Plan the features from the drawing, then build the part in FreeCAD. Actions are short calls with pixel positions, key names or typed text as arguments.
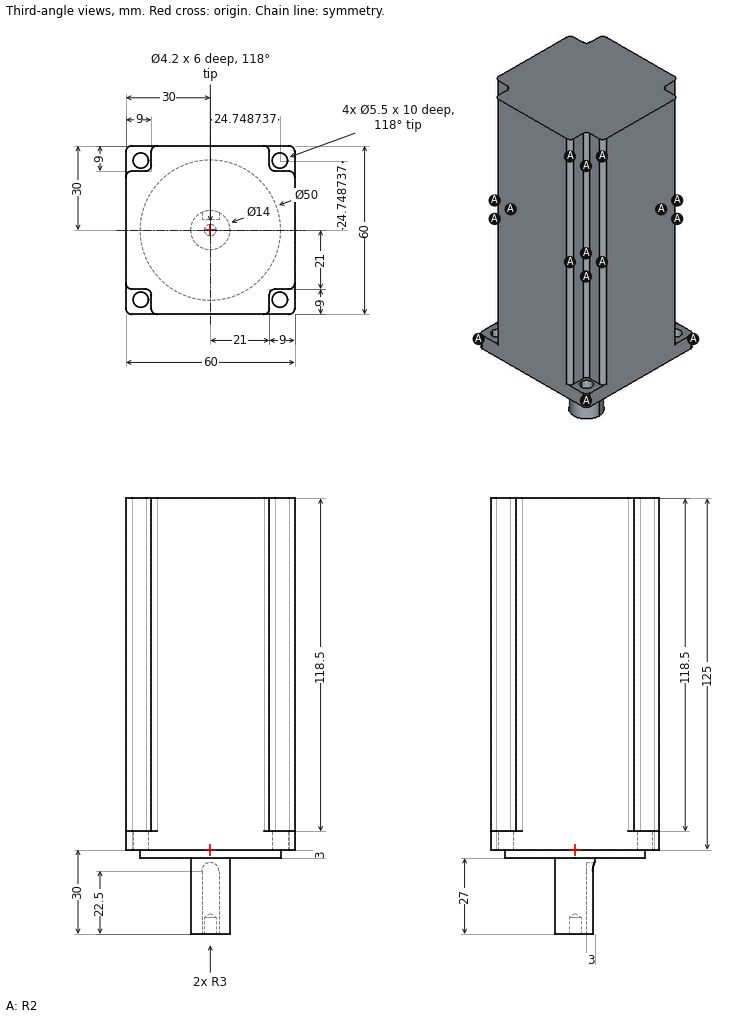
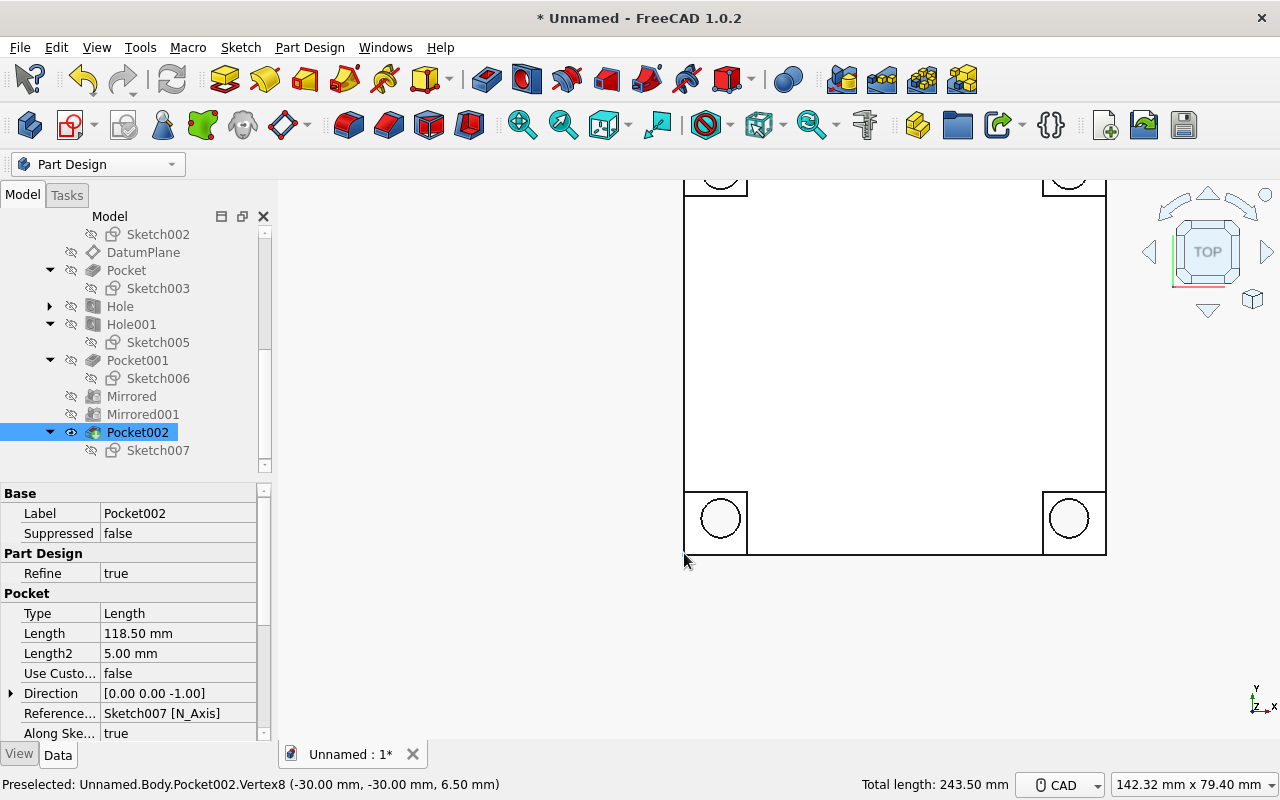
click(524, 126)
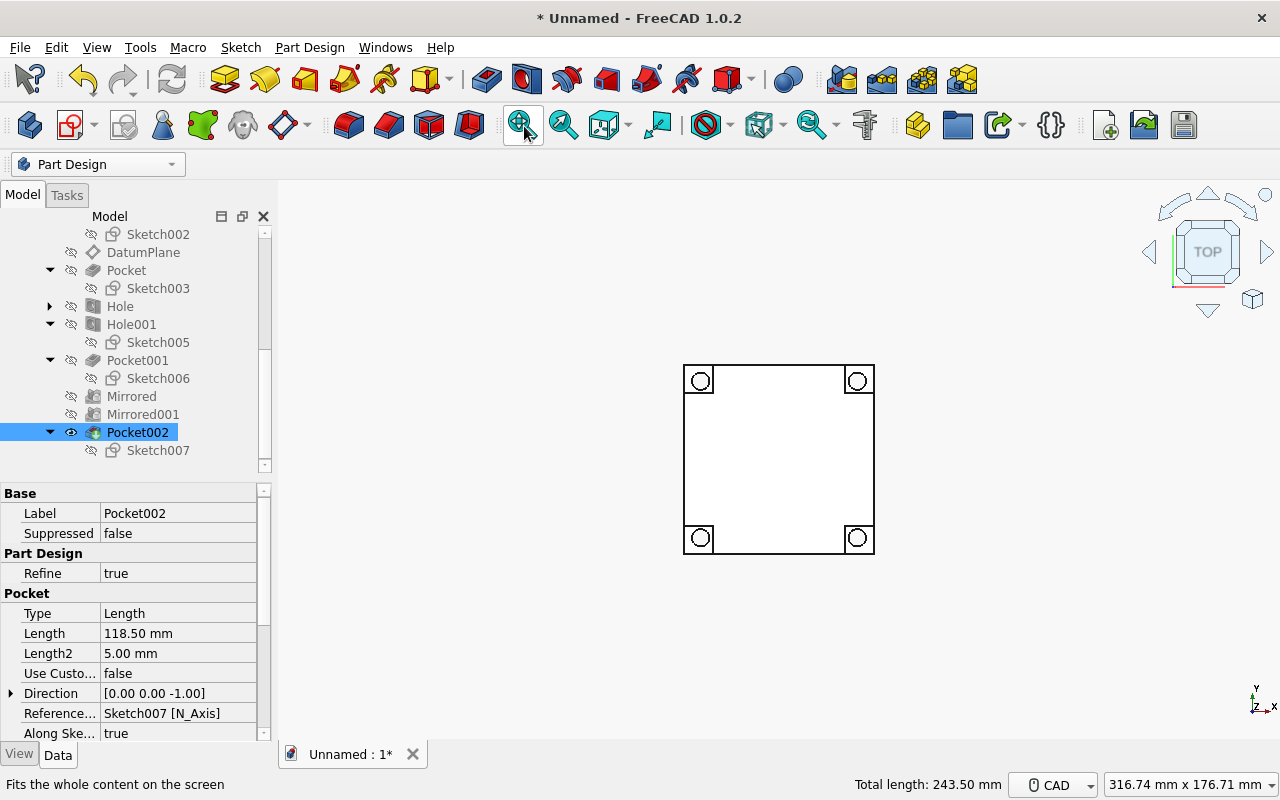
key(0)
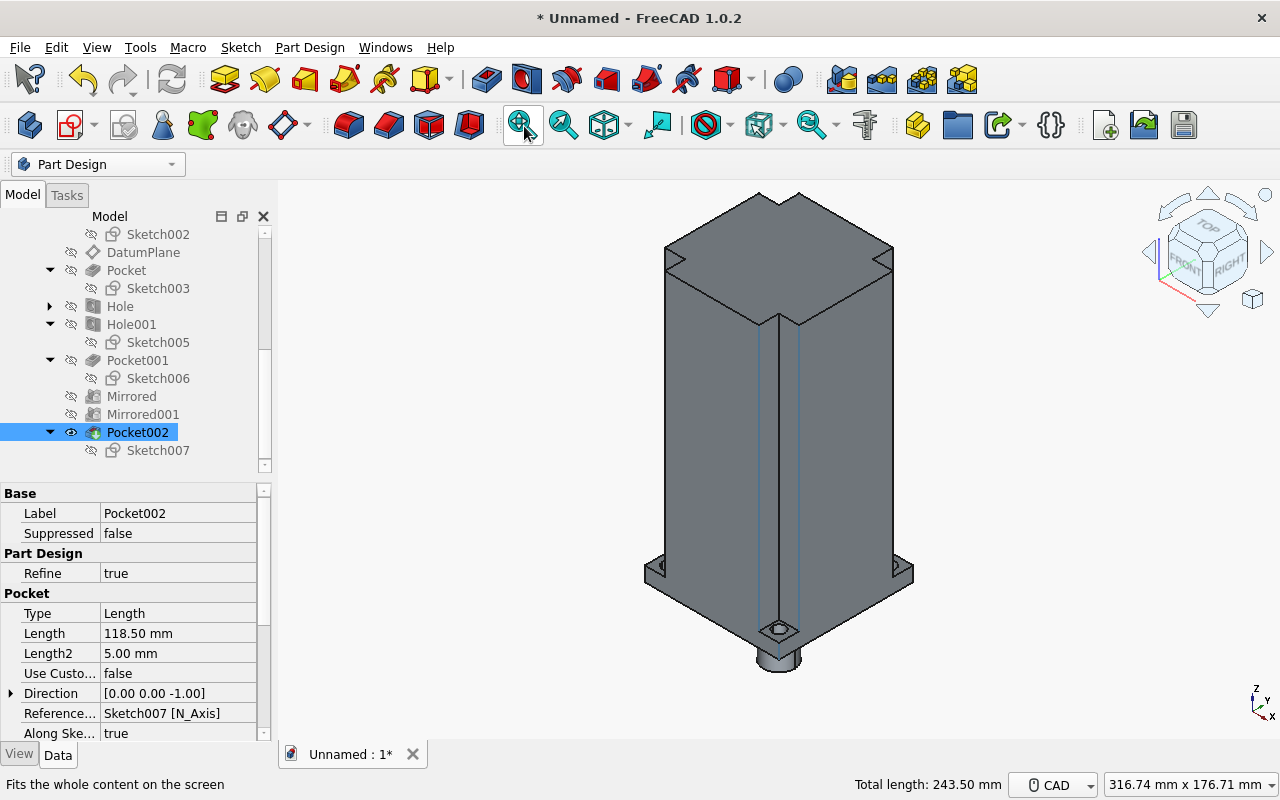
scroll(645, 573, up, 4)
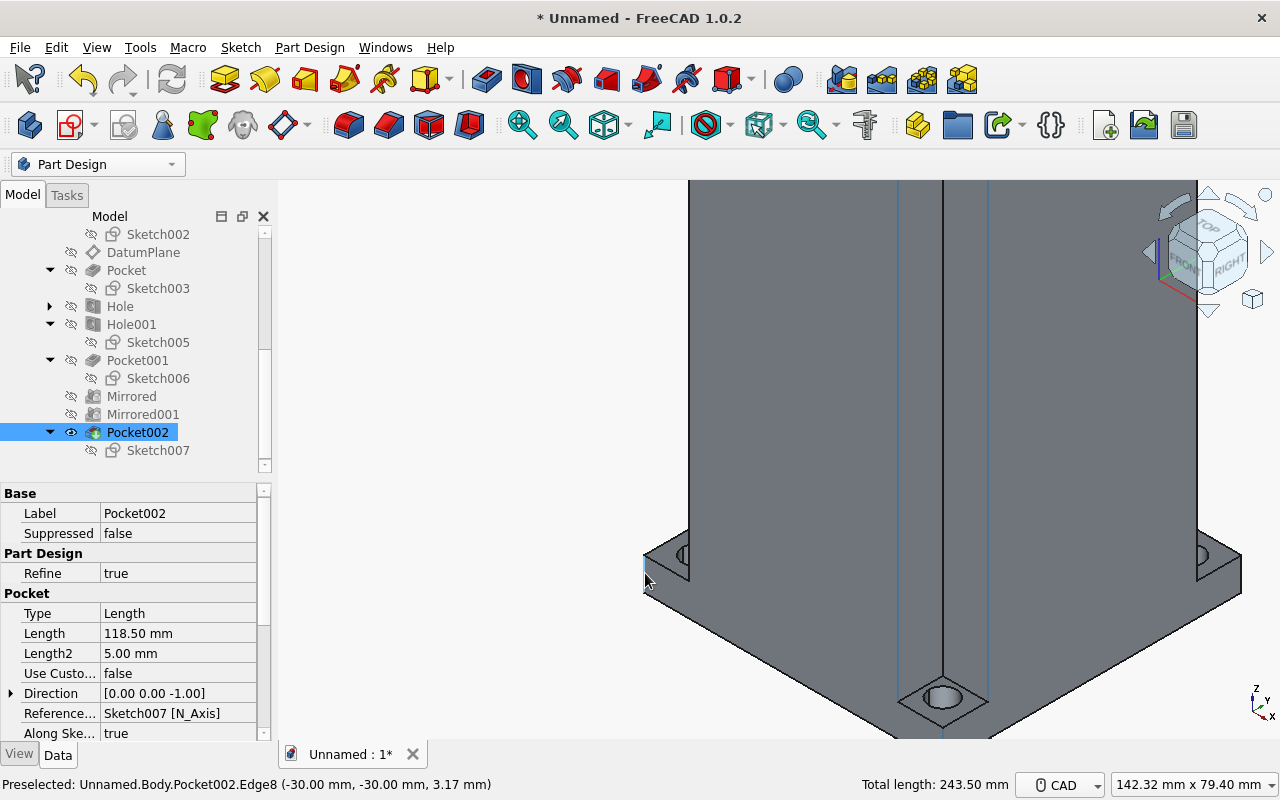
click(524, 126)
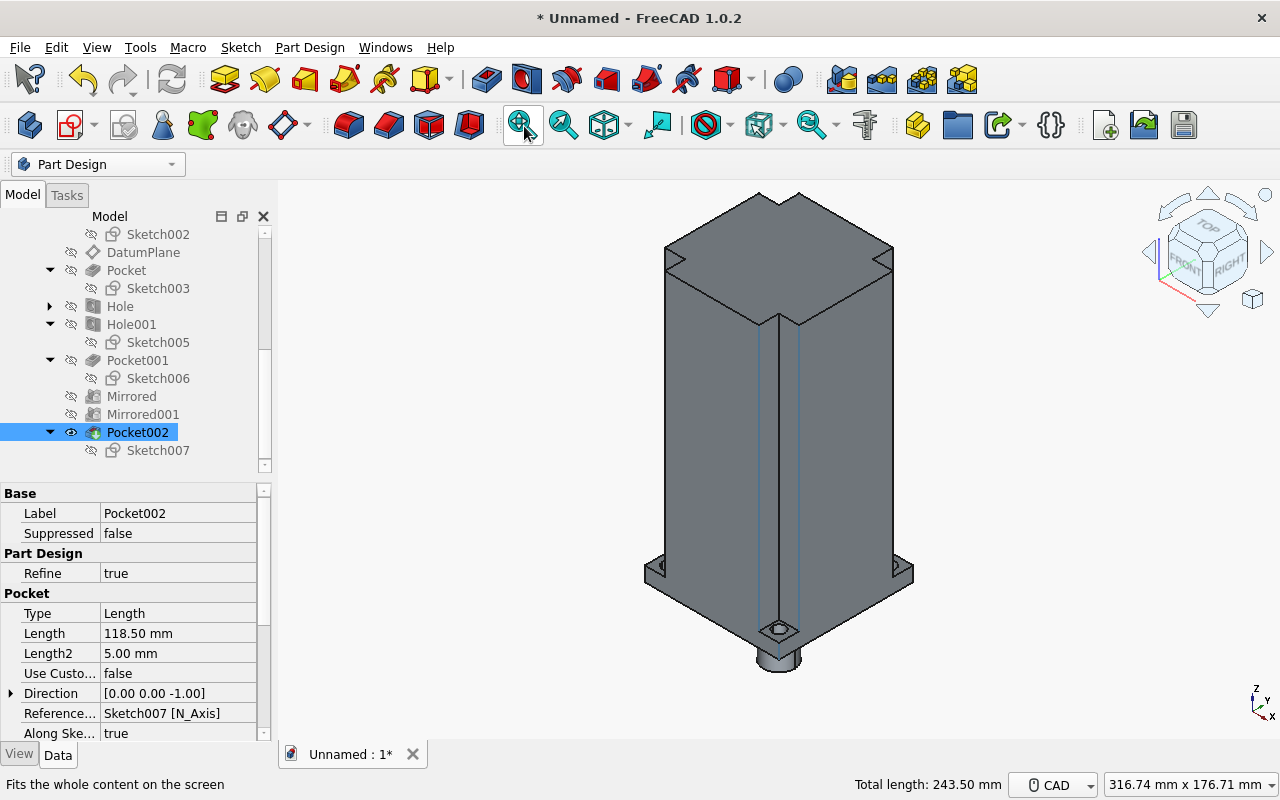
key(1)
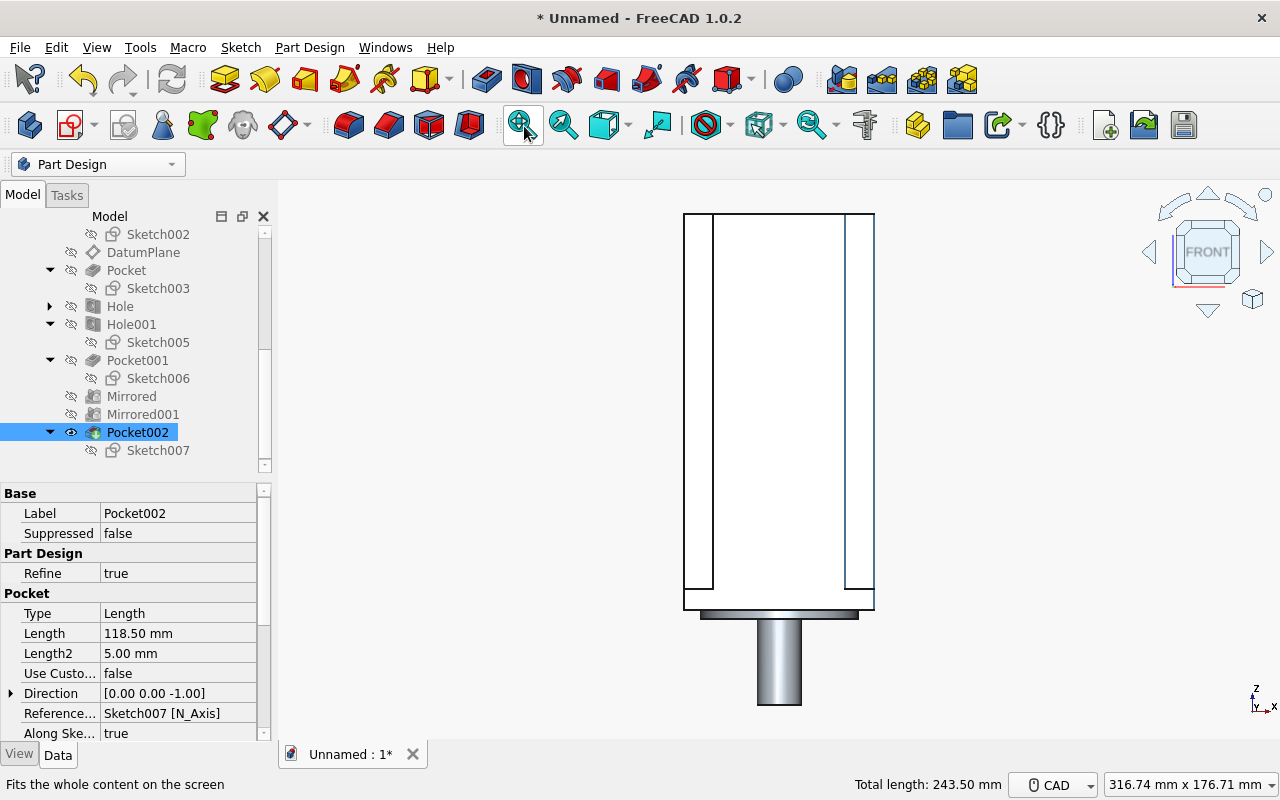
click(684, 598, ctrl)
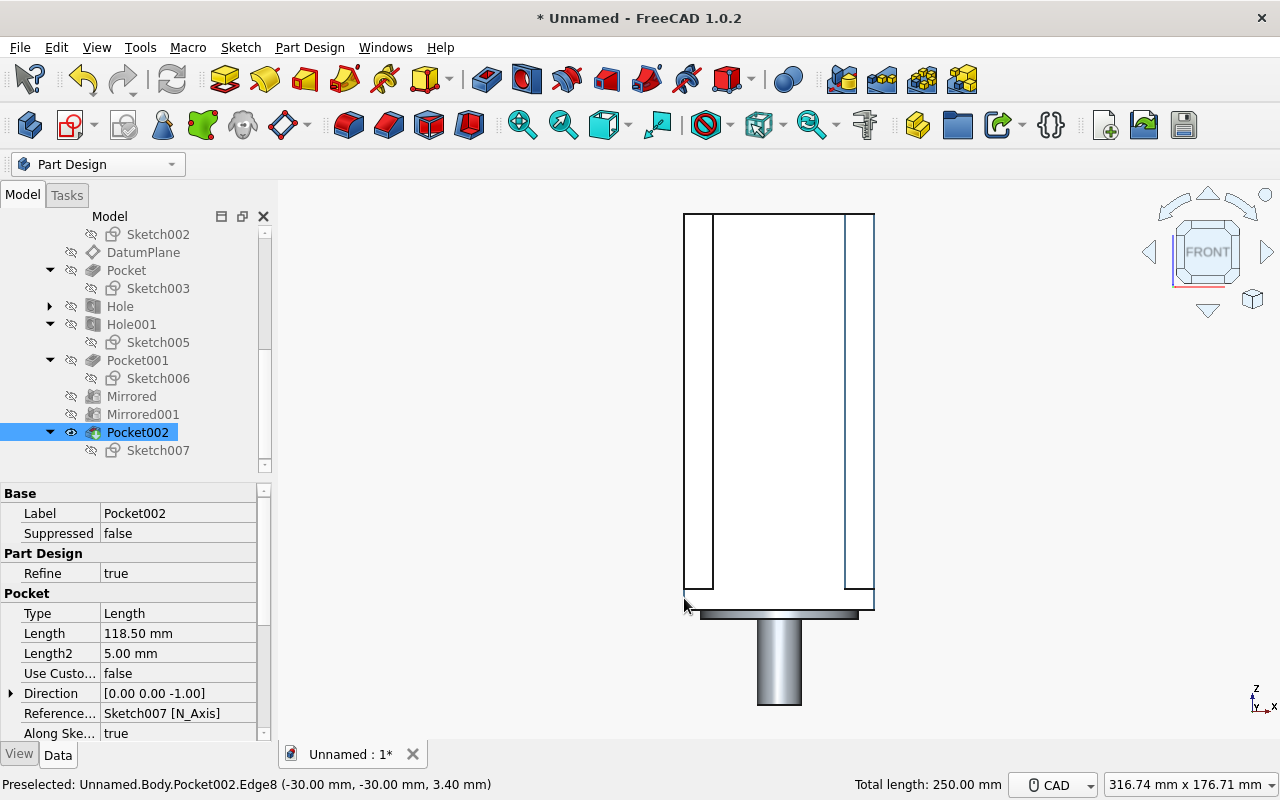
click(684, 401, ctrl)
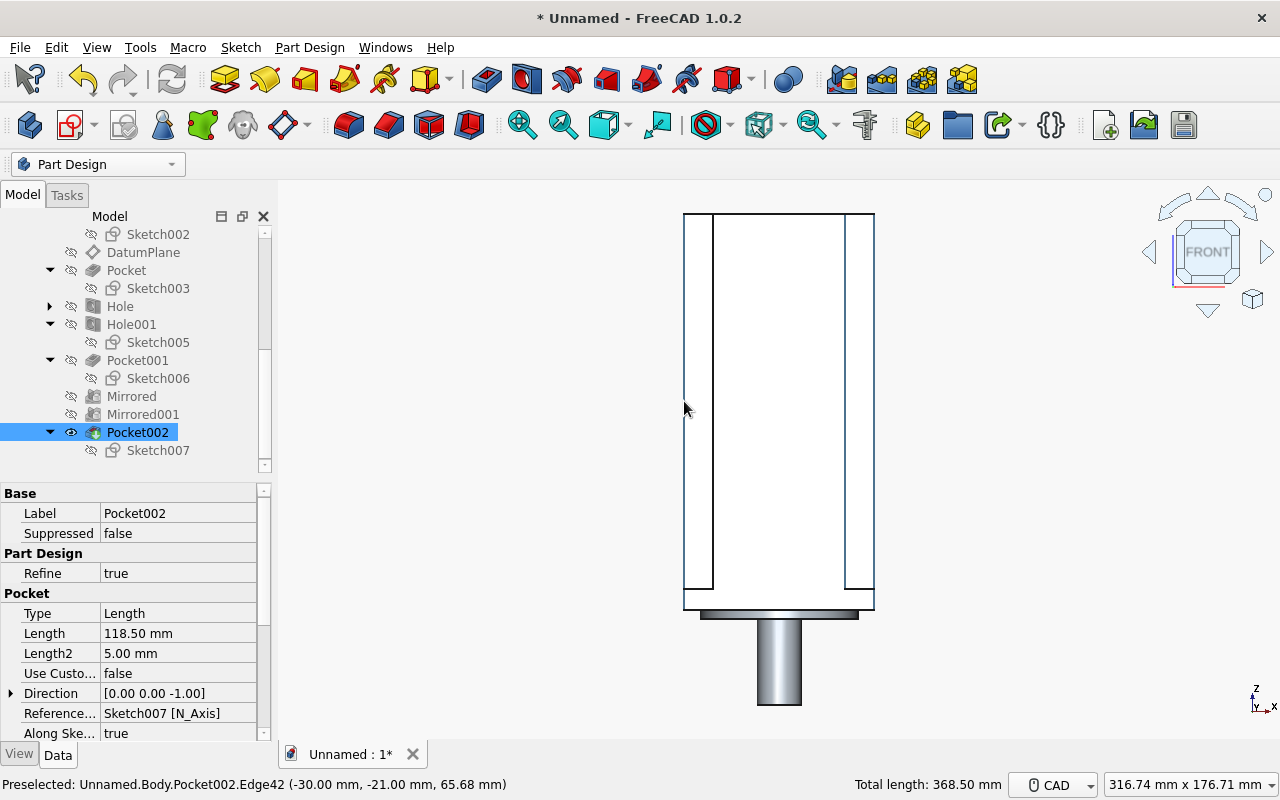
click(713, 401, ctrl)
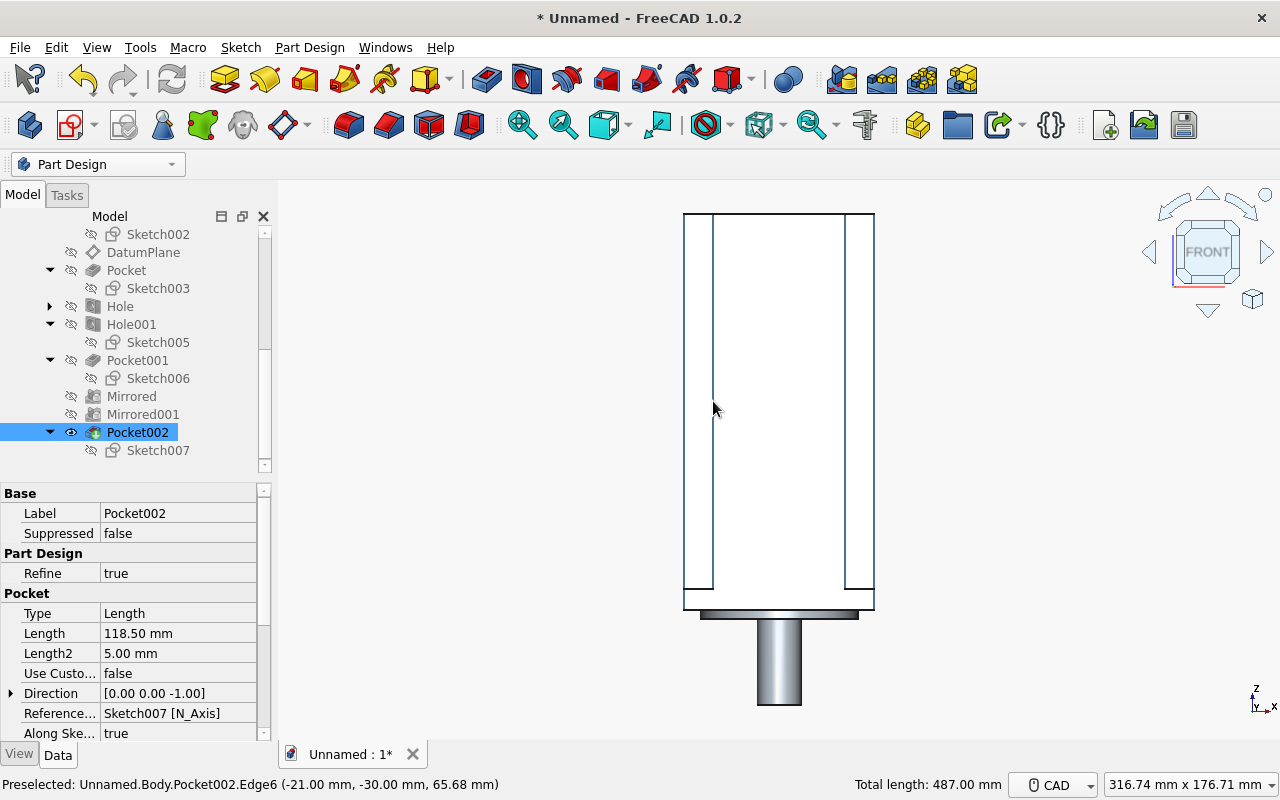
key(3)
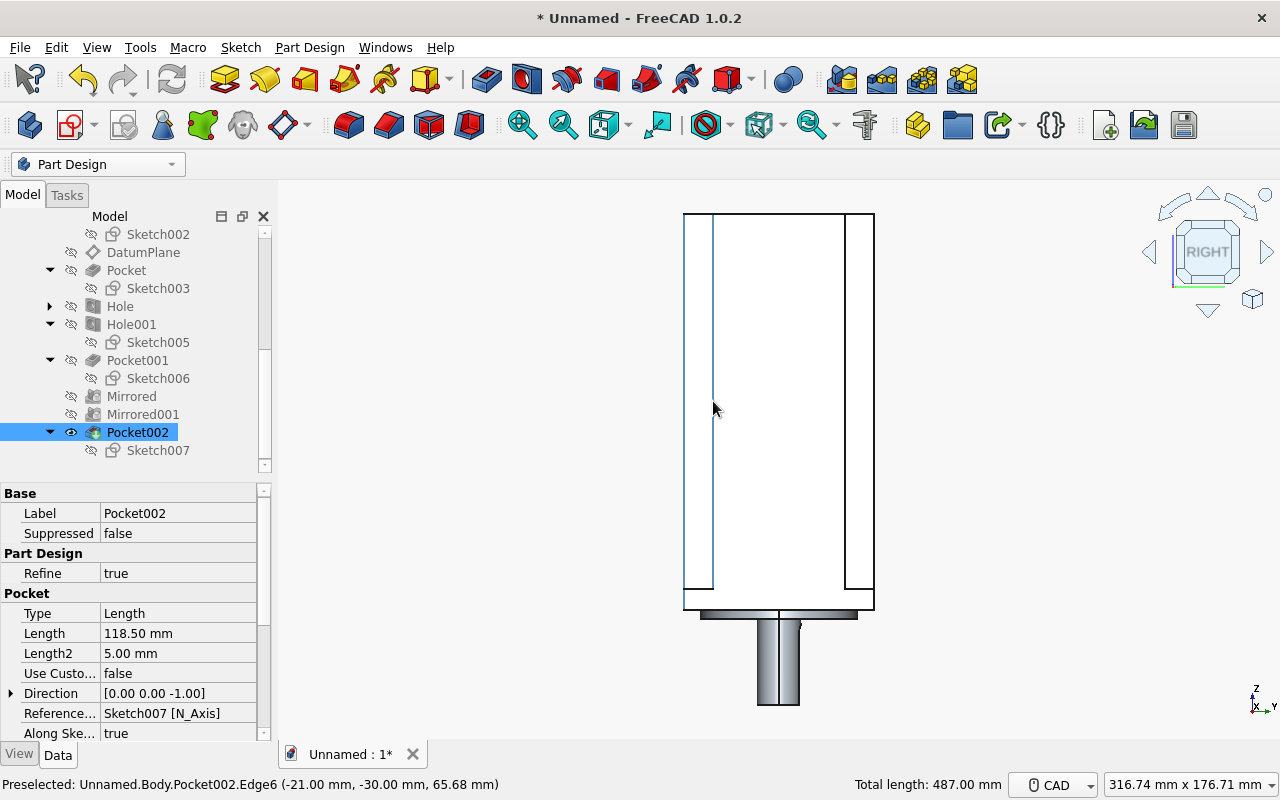
click(874, 598, ctrl)